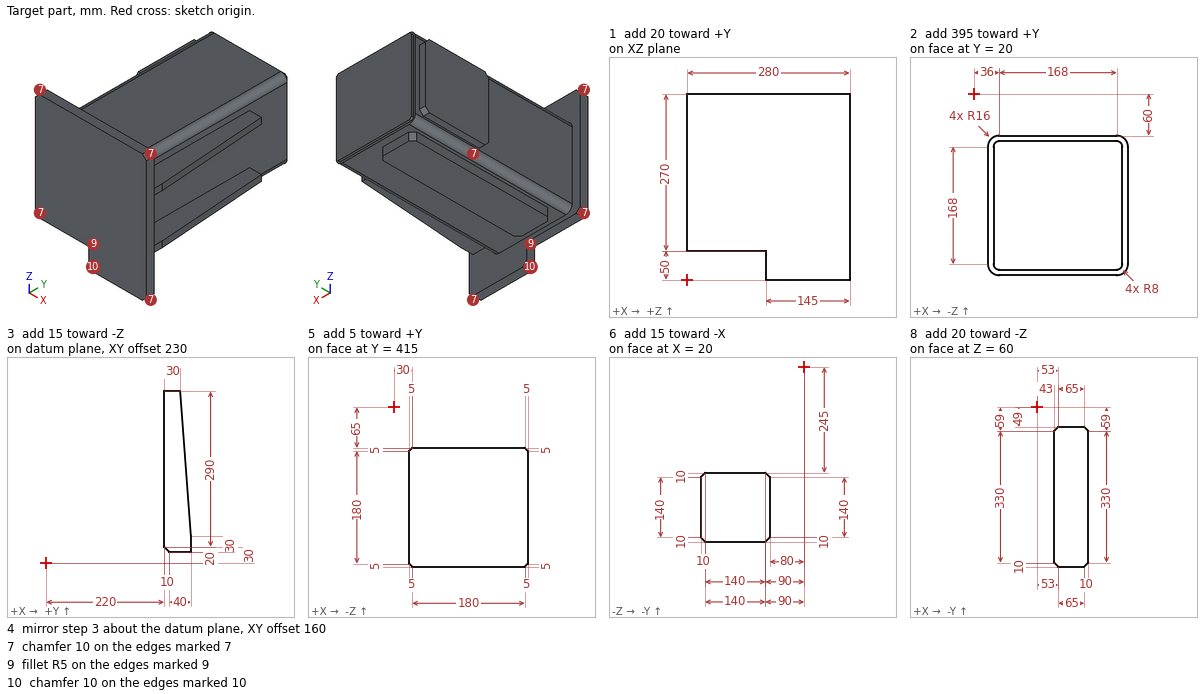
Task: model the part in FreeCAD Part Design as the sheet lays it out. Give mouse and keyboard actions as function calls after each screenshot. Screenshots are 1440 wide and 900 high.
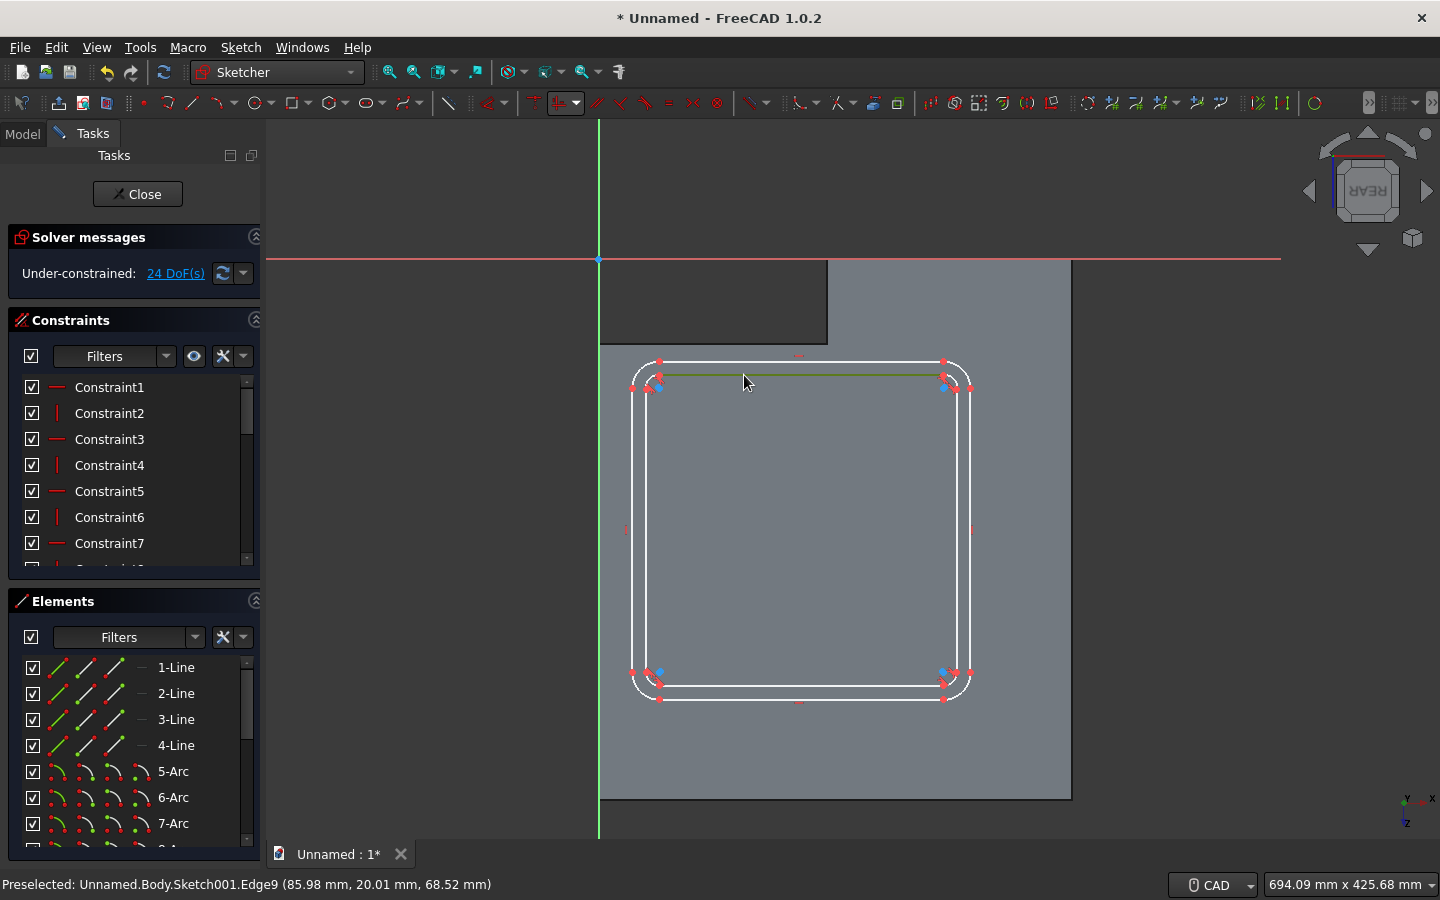
scroll(954, 379, up, 2)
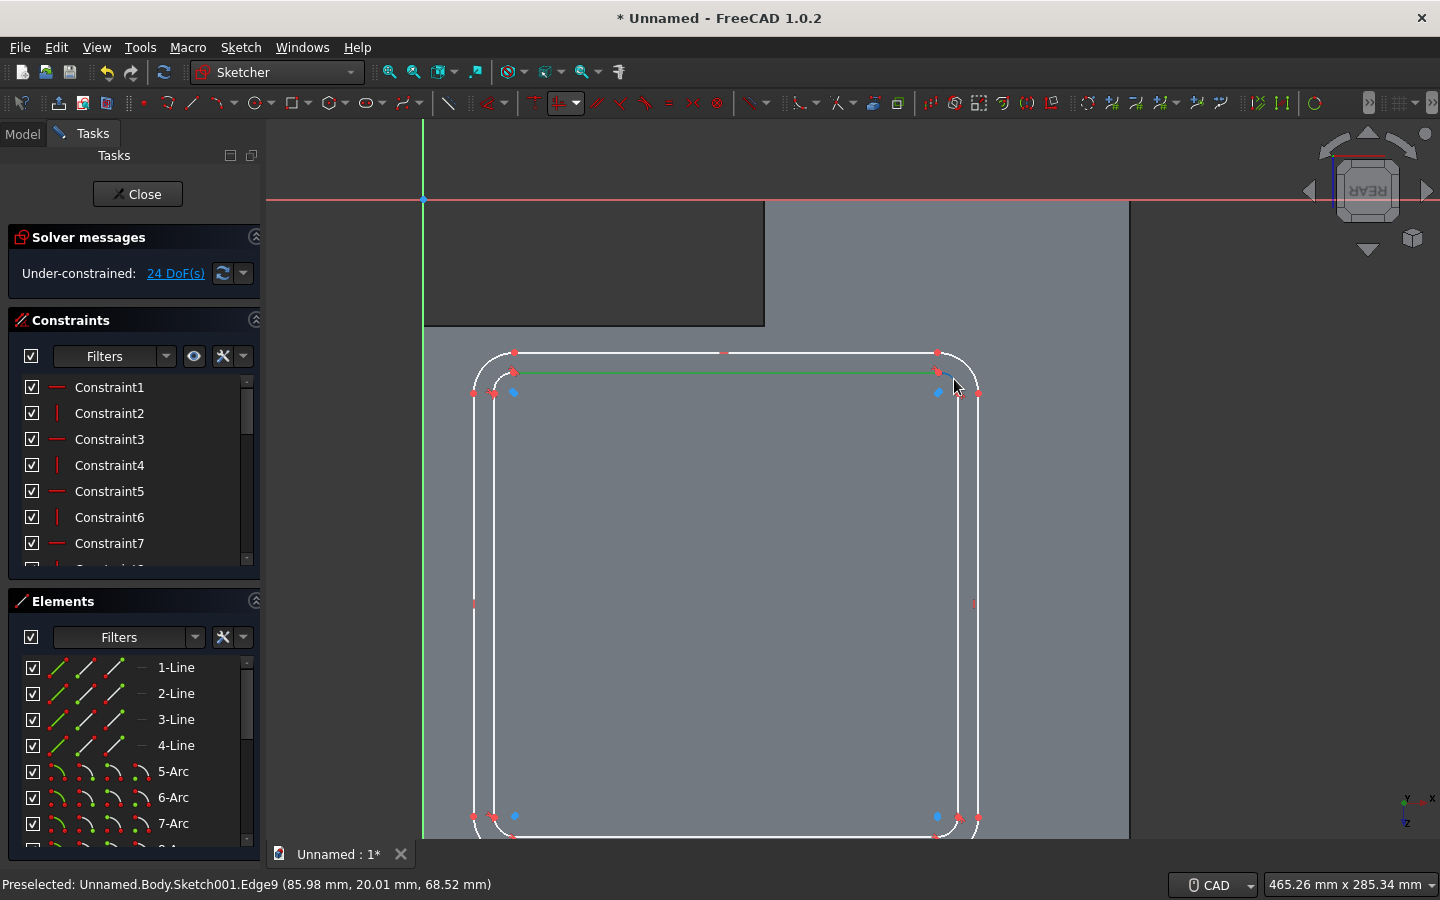
click(953, 379)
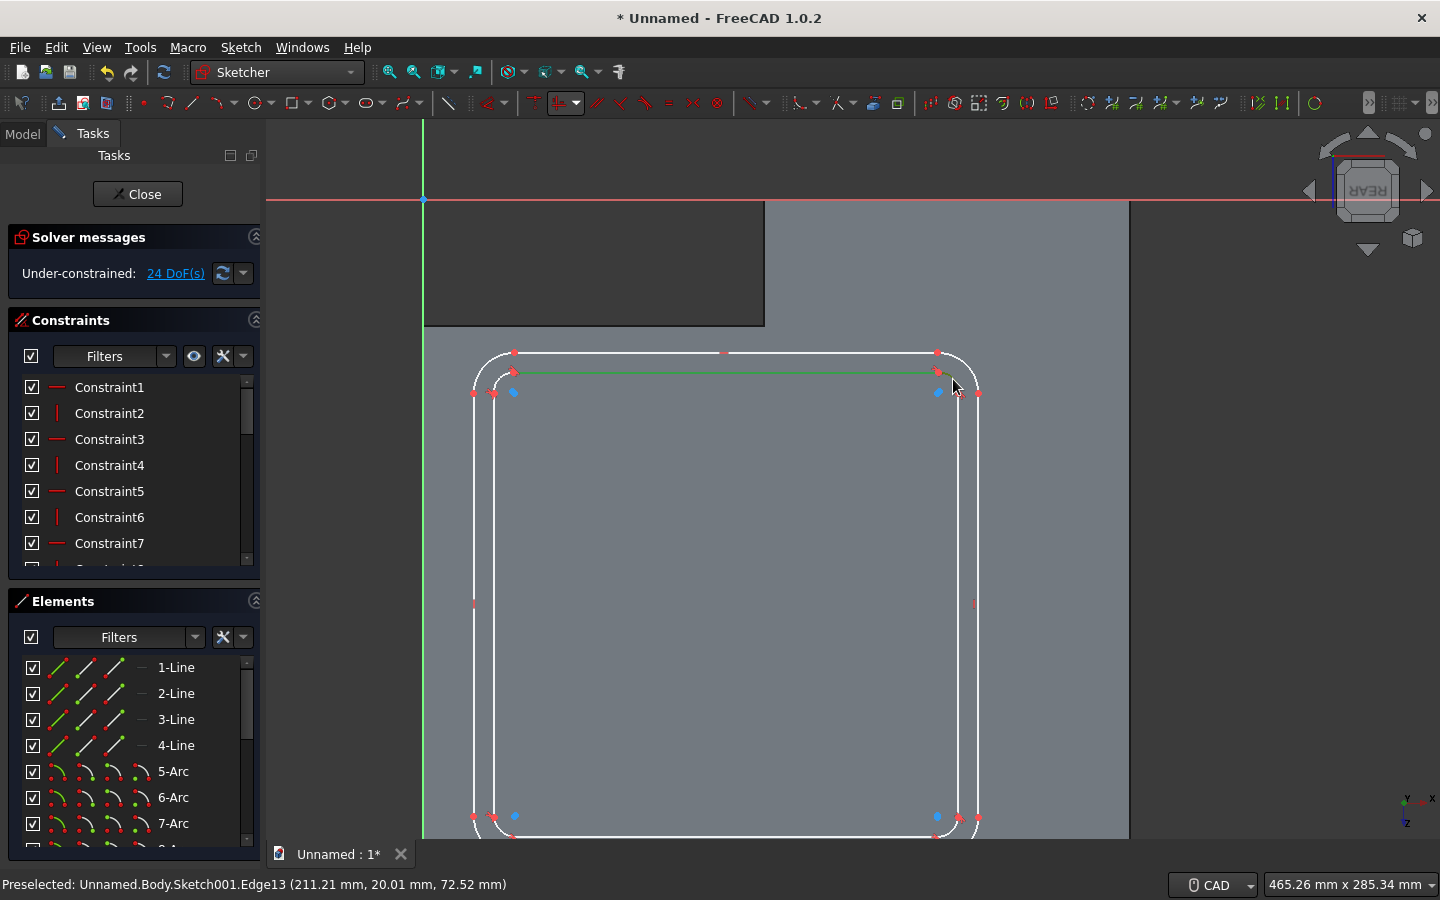
click(646, 104)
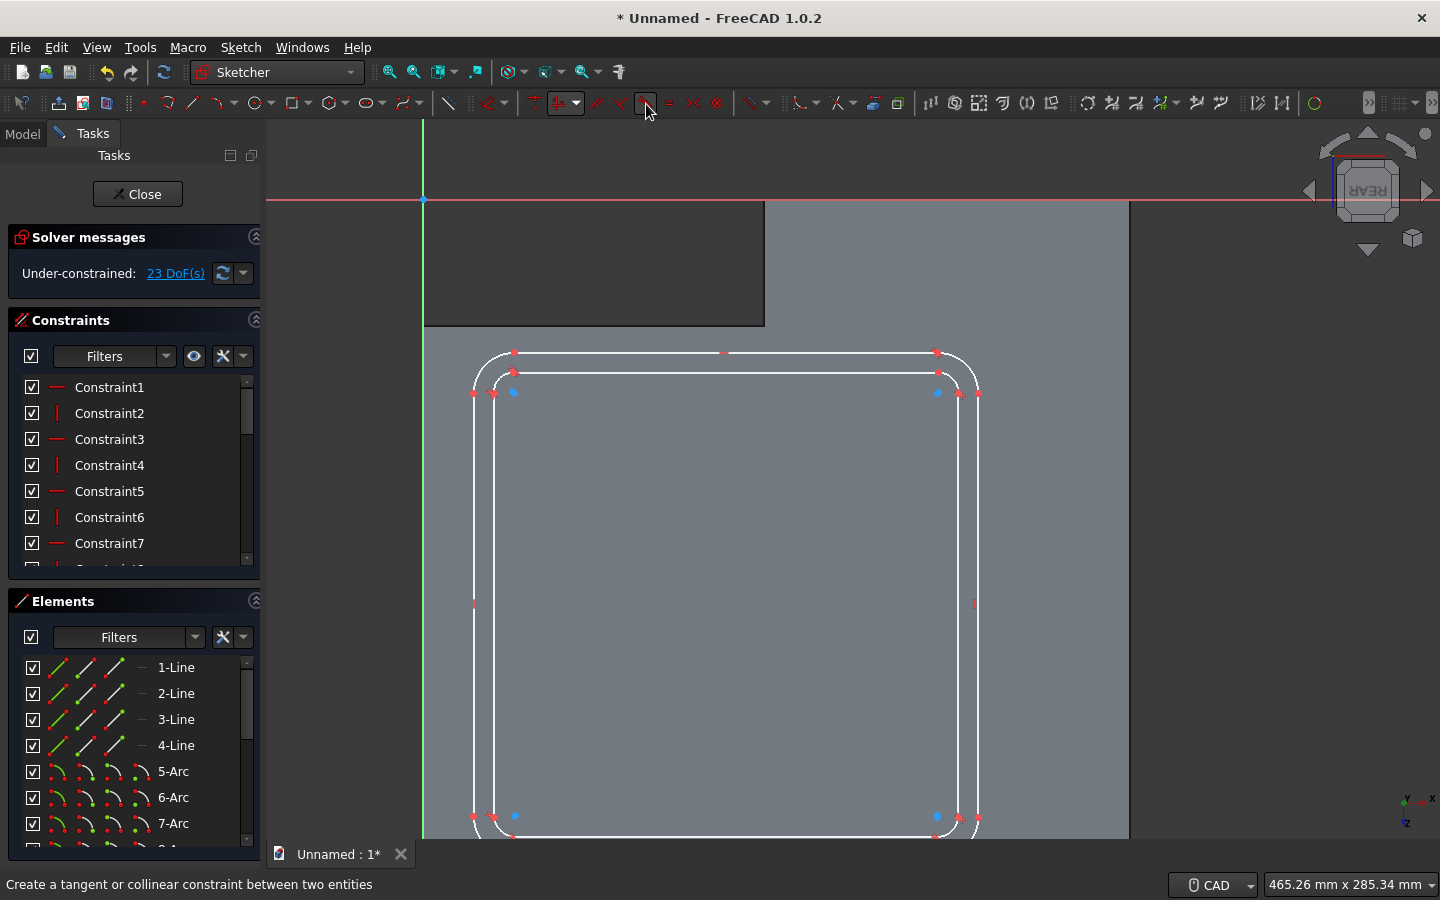
click(641, 373)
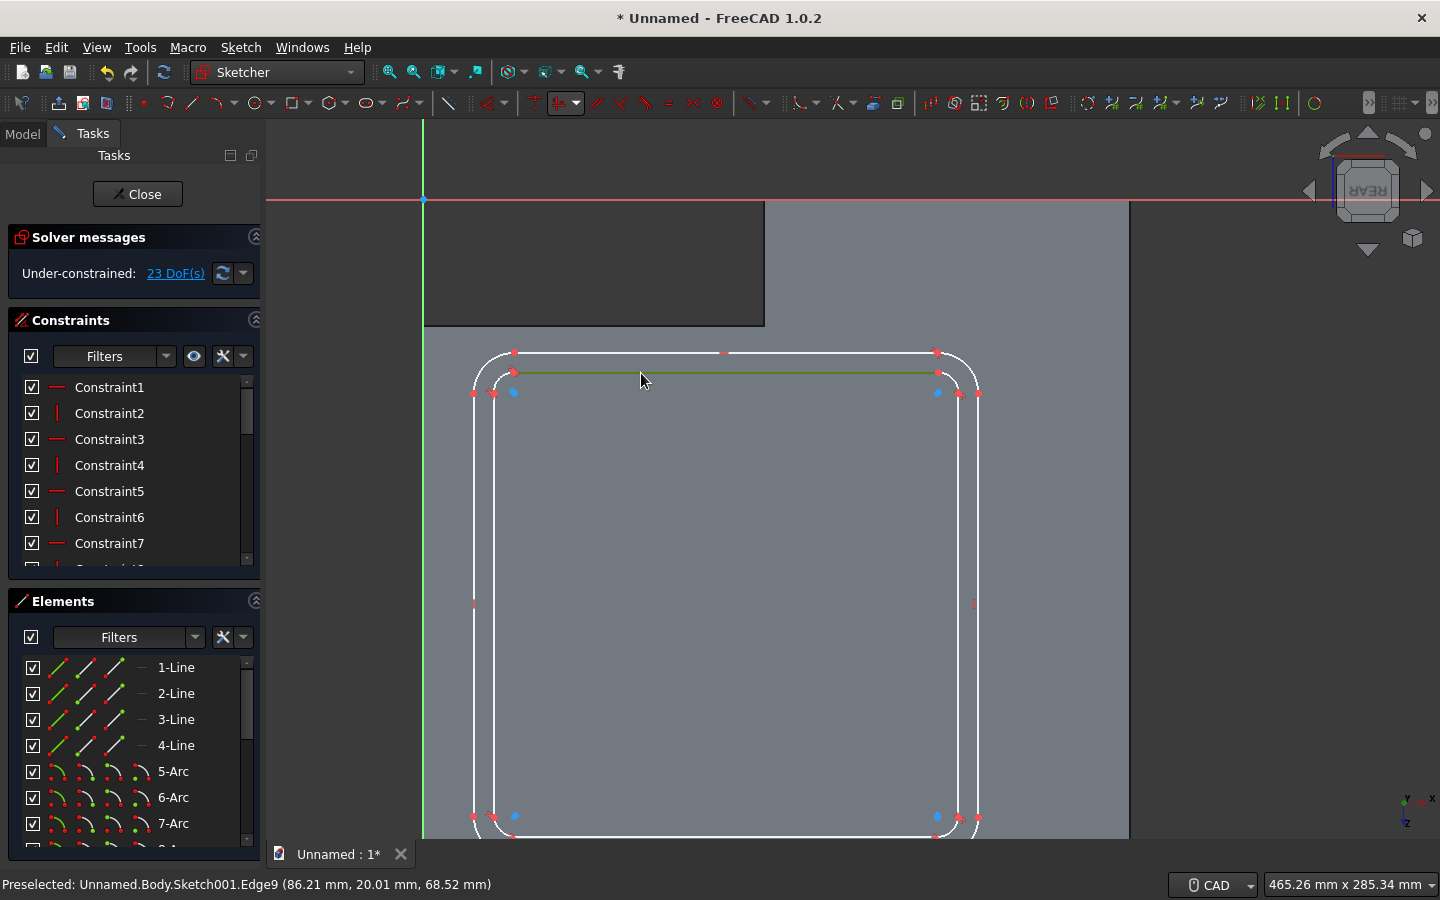
scroll(504, 375, up, 2)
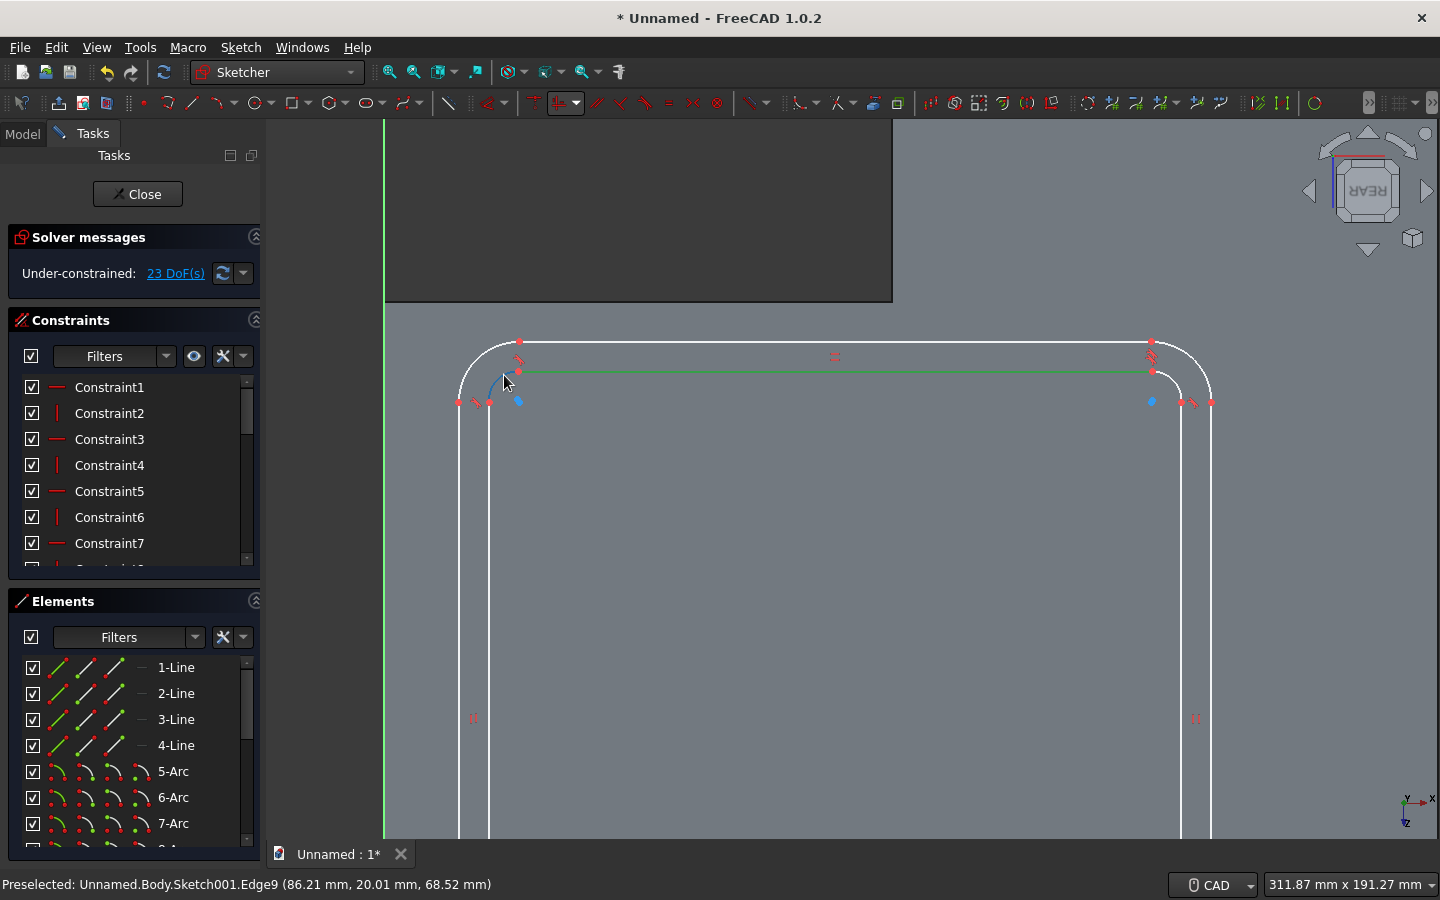
click(504, 375)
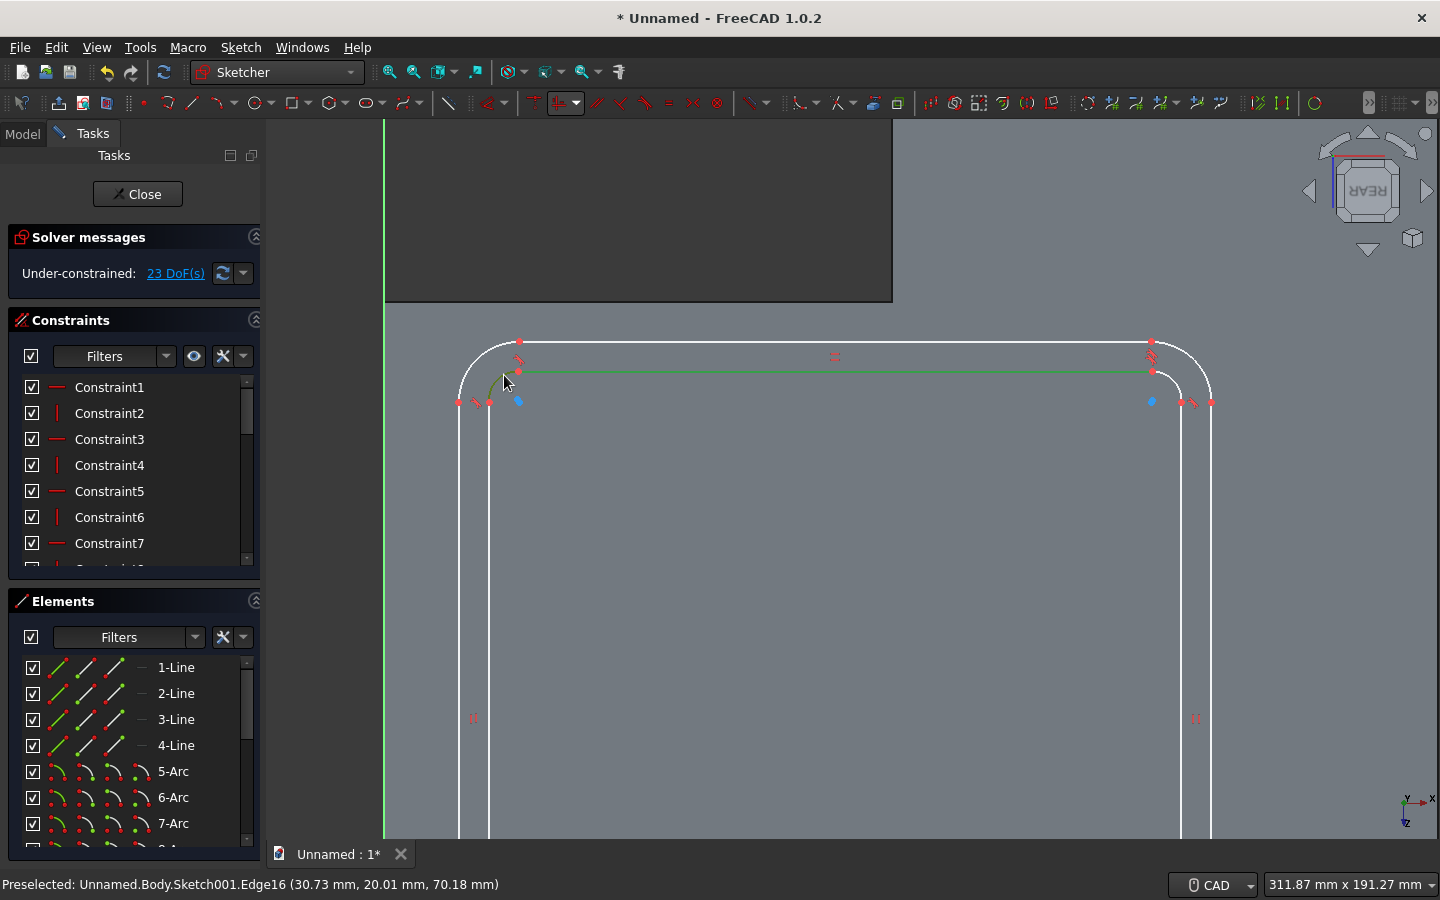
click(646, 104)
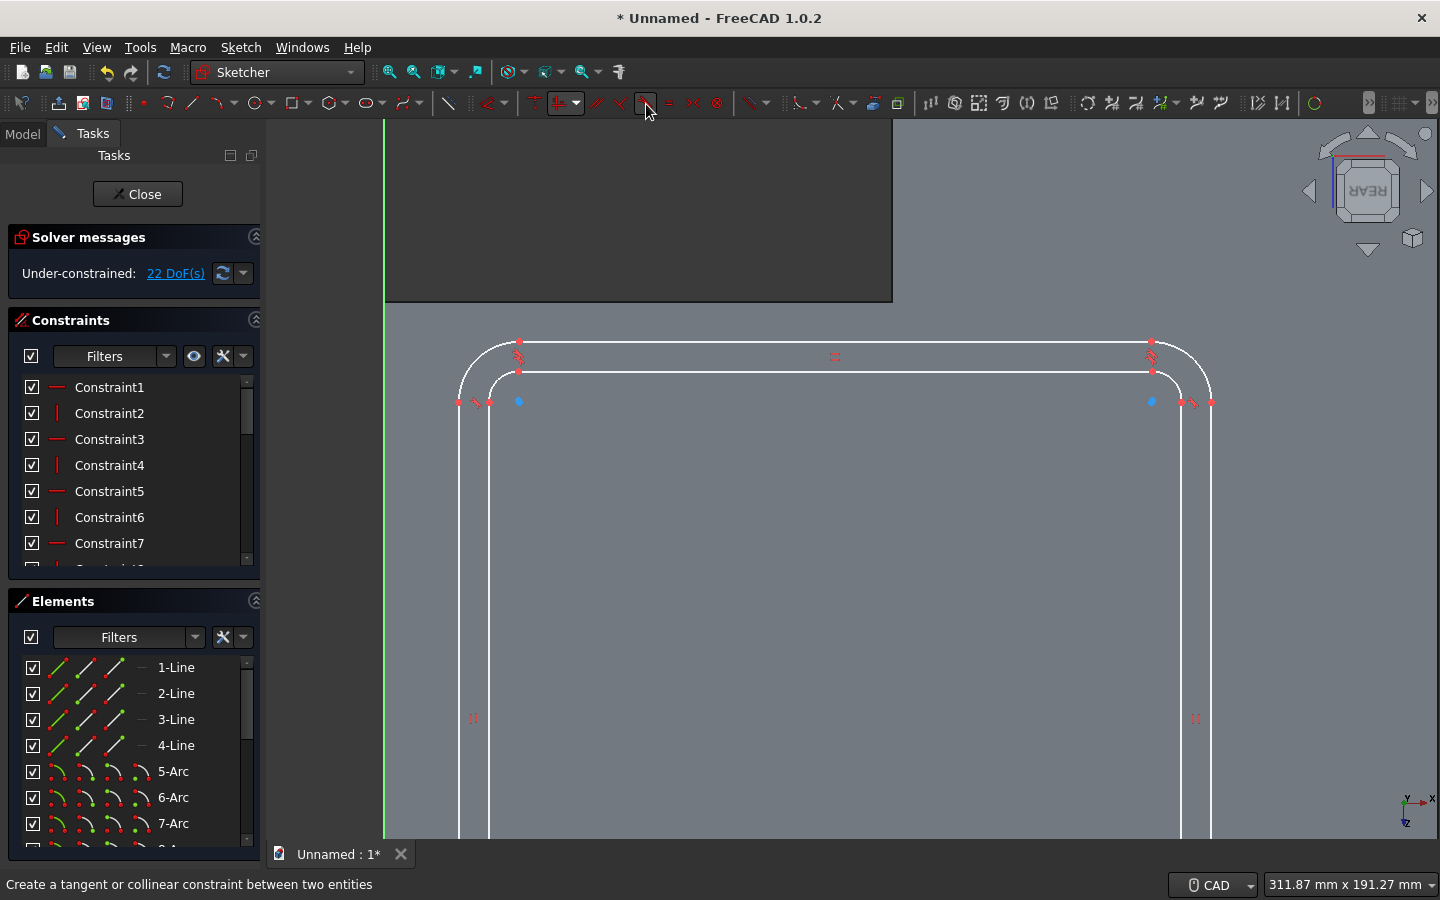
click(1181, 592)